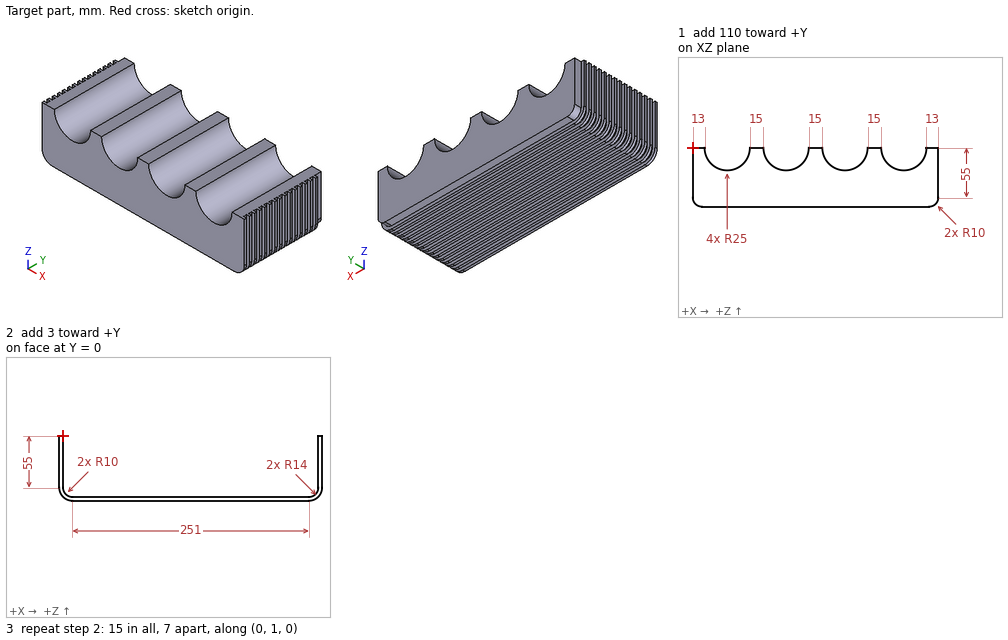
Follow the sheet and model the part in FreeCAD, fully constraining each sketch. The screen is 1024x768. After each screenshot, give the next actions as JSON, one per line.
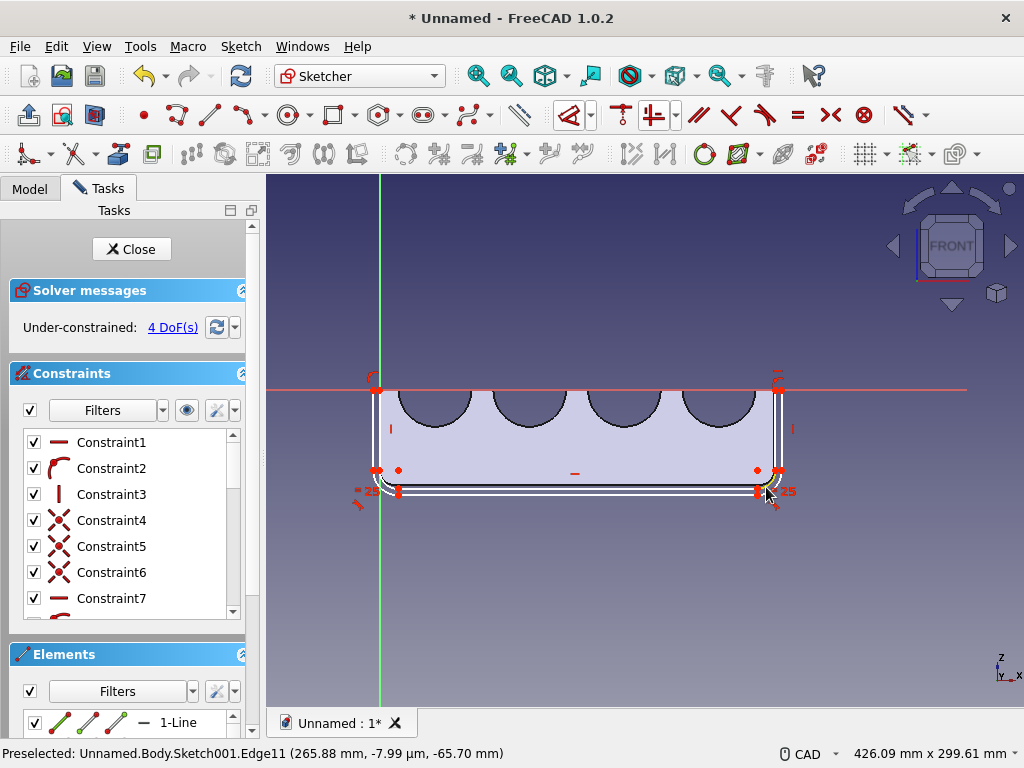
{"action": "scroll", "coordinate": [387, 493], "scroll_direction": "up", "scroll_amount": 4}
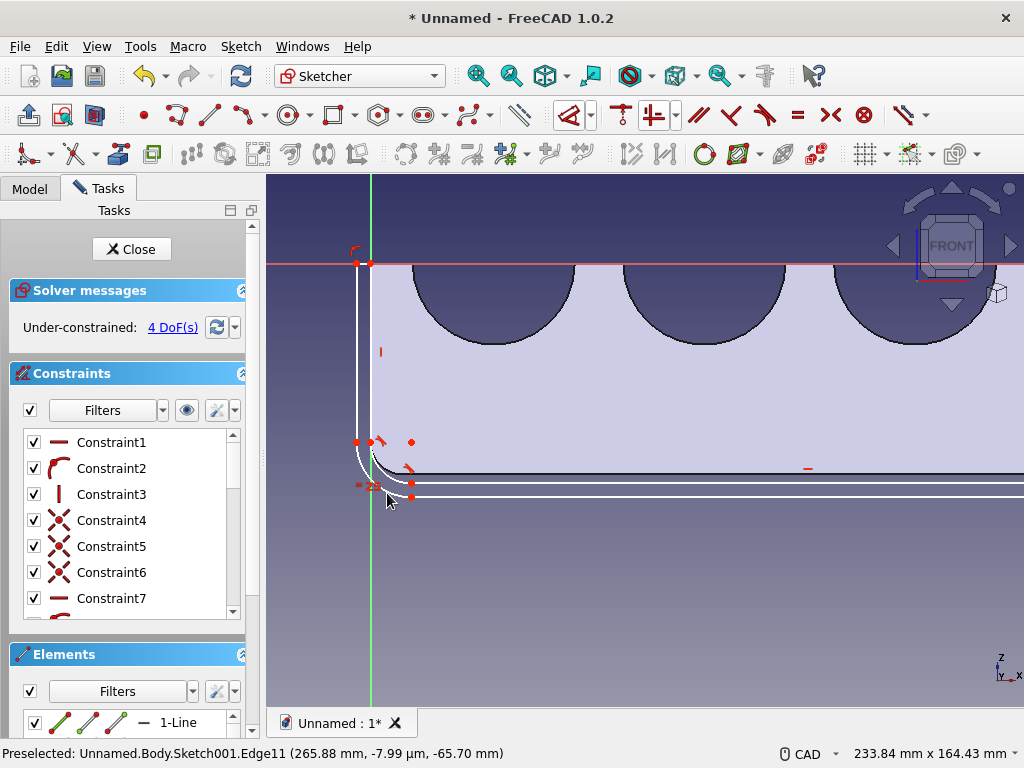
{"action": "left_click", "coordinate": [387, 491]}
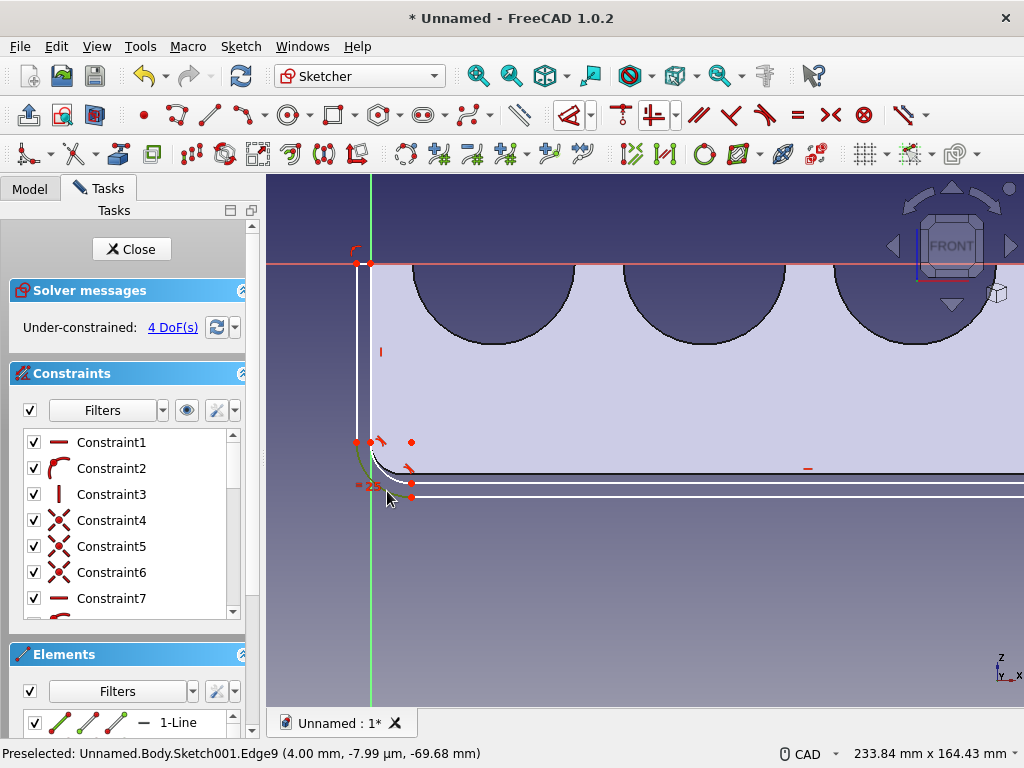
{"action": "key", "text": "k r"}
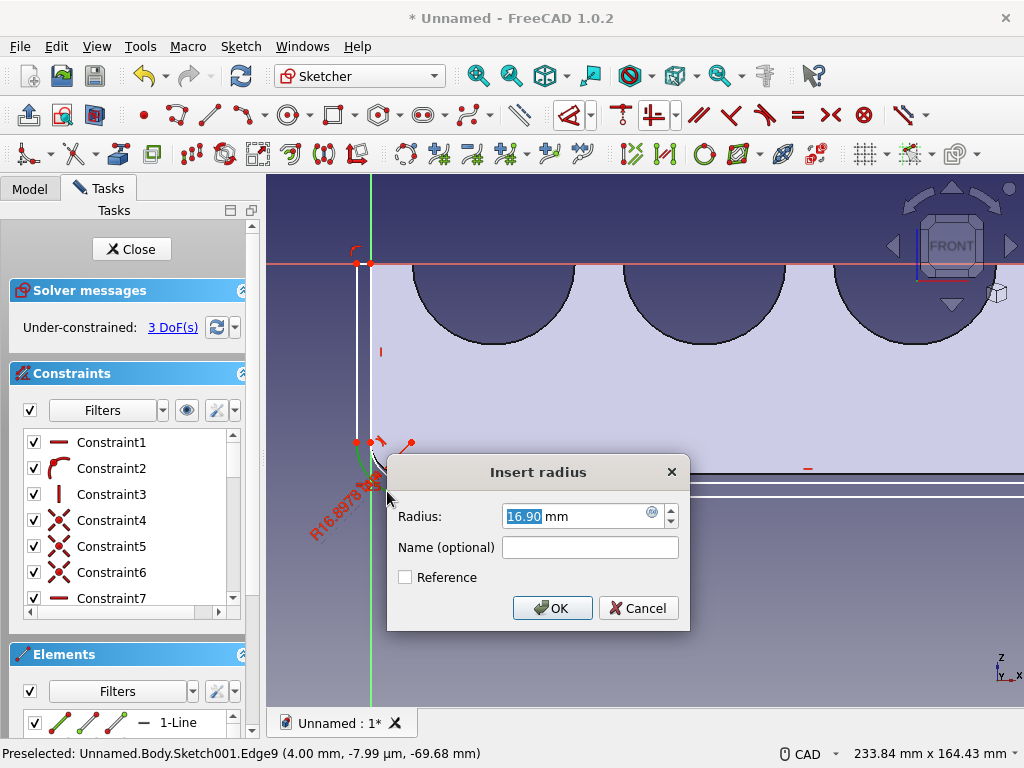
{"action": "type", "text": "14"}
{"action": "key", "text": "Return"}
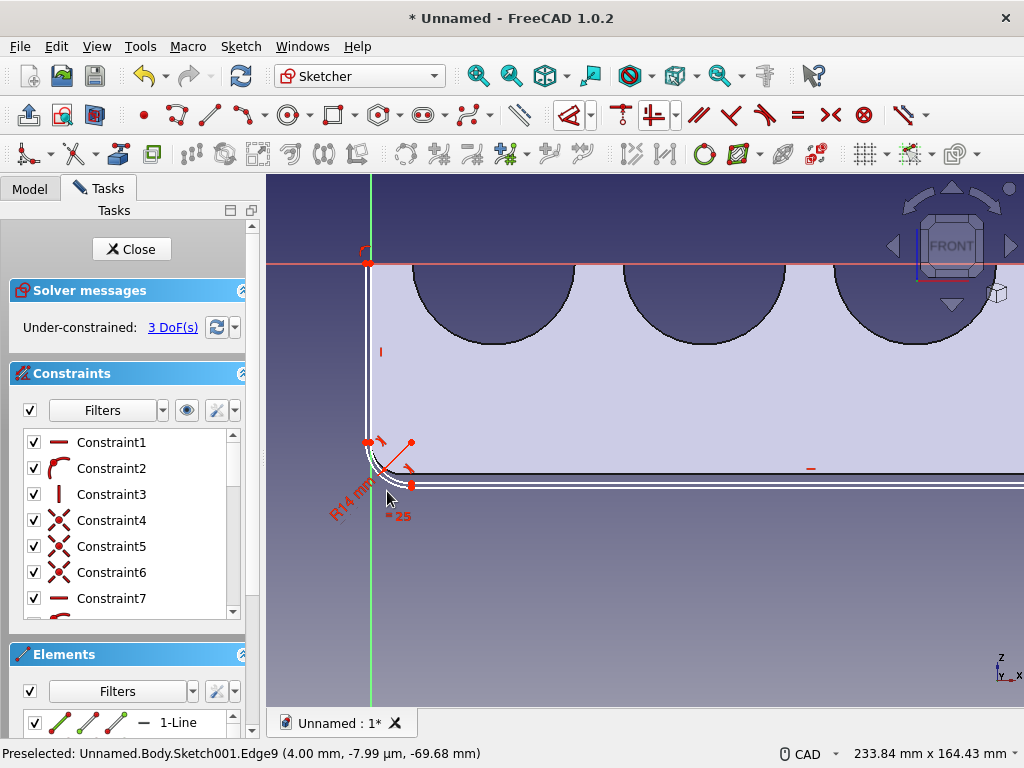
{"action": "scroll", "coordinate": [373, 455], "scroll_direction": "up", "scroll_amount": 6}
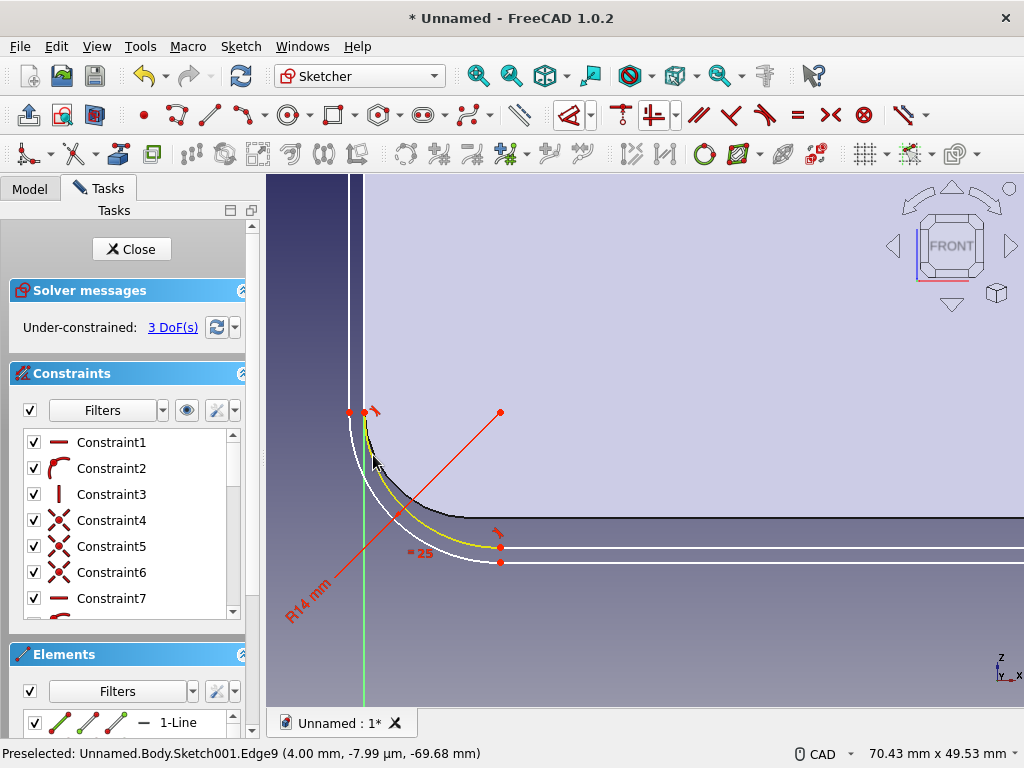
{"action": "left_click", "coordinate": [371, 454]}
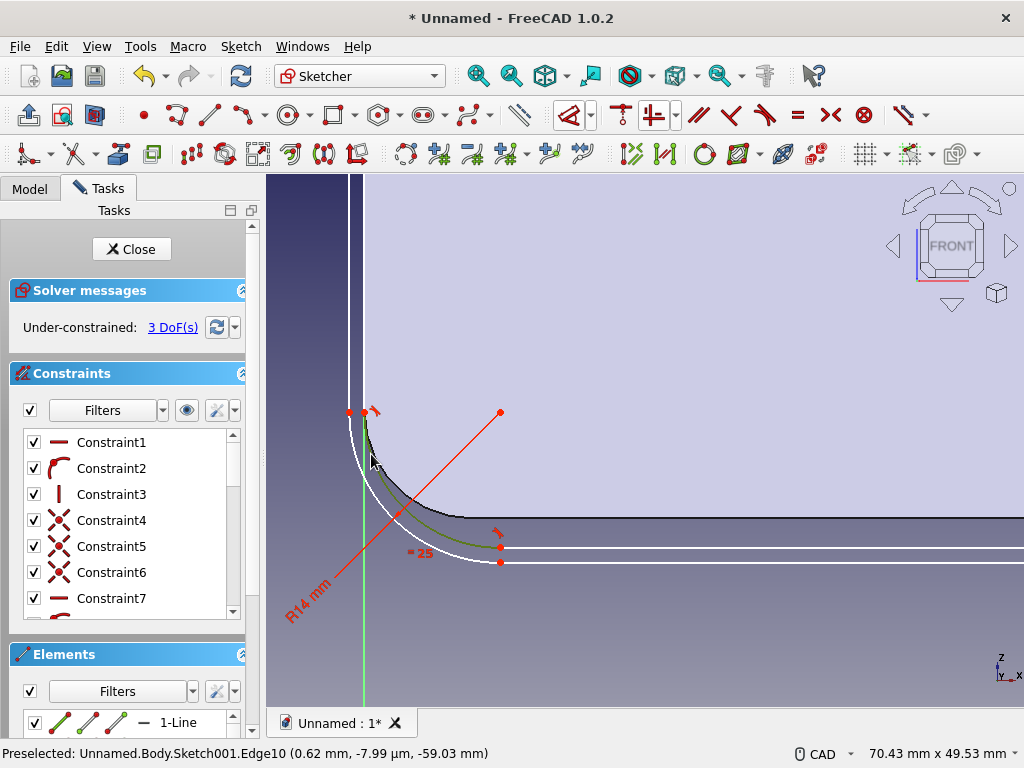
{"action": "key", "text": "k r"}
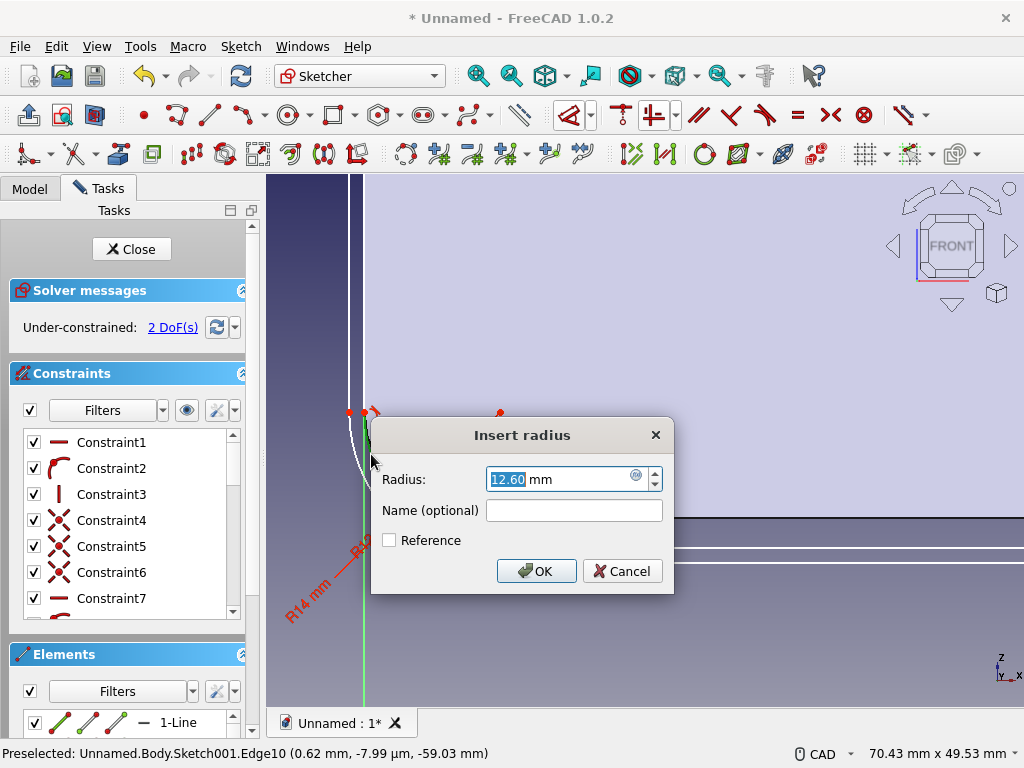
{"action": "type", "text": "10"}
{"action": "key", "text": "Return"}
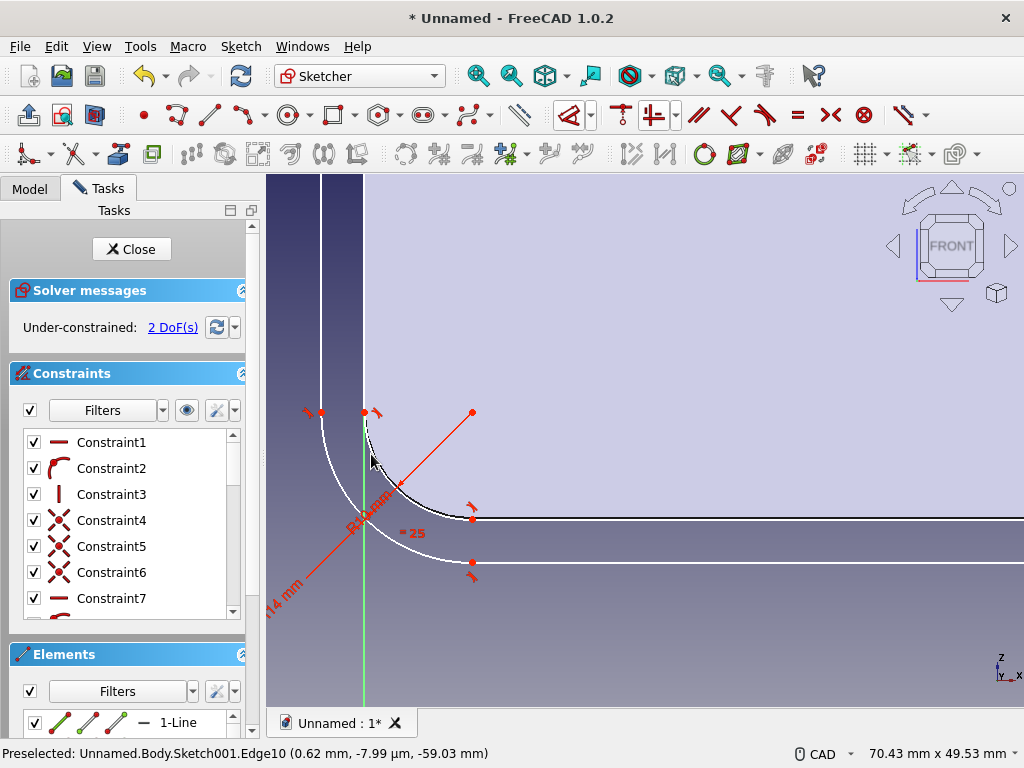
{"action": "scroll", "coordinate": [381, 480], "scroll_direction": "down", "scroll_amount": 10}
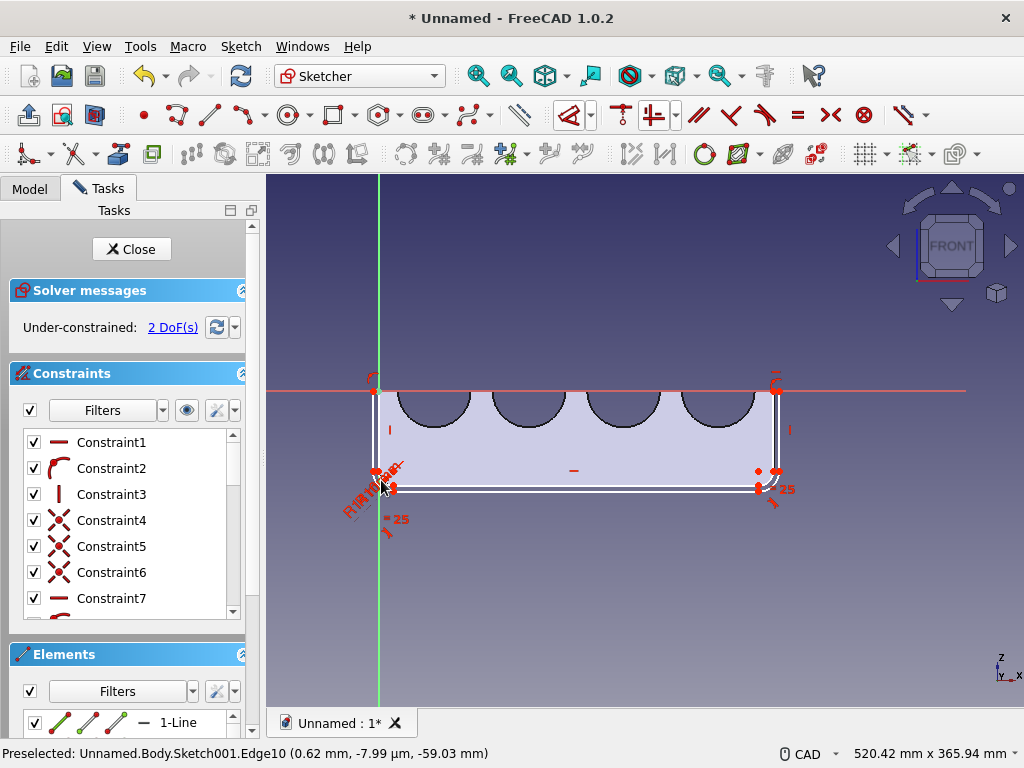
{"action": "scroll", "coordinate": [373, 447], "scroll_direction": "up", "scroll_amount": 5}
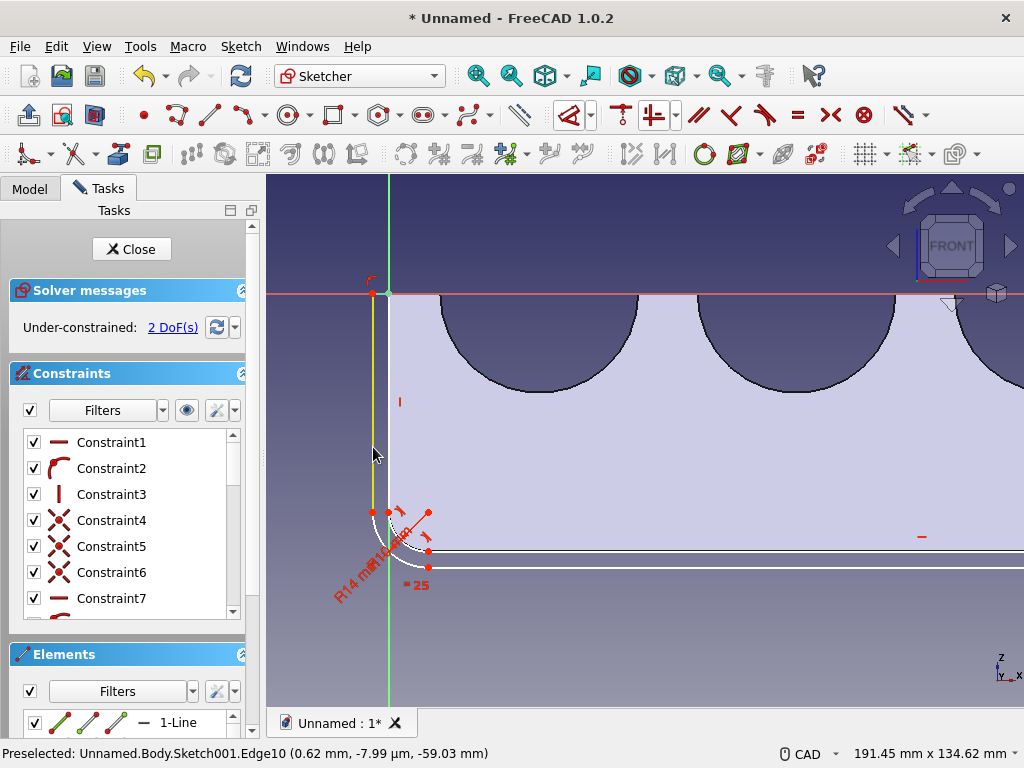
{"action": "left_click", "coordinate": [373, 447]}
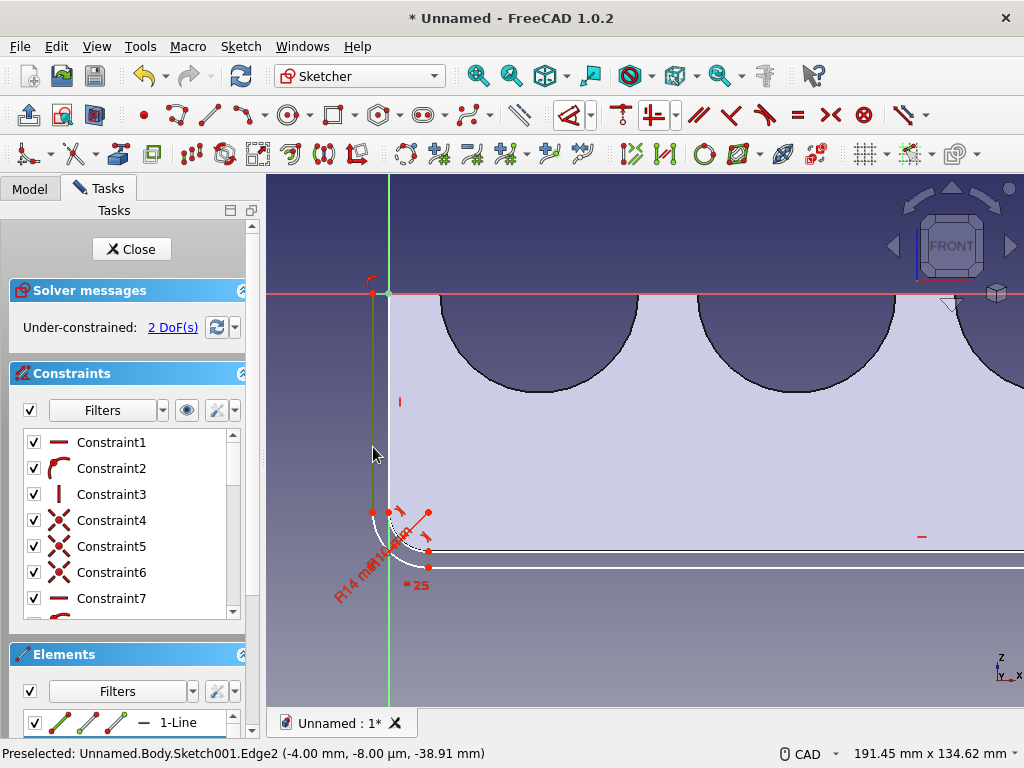
{"action": "key", "text": "i"}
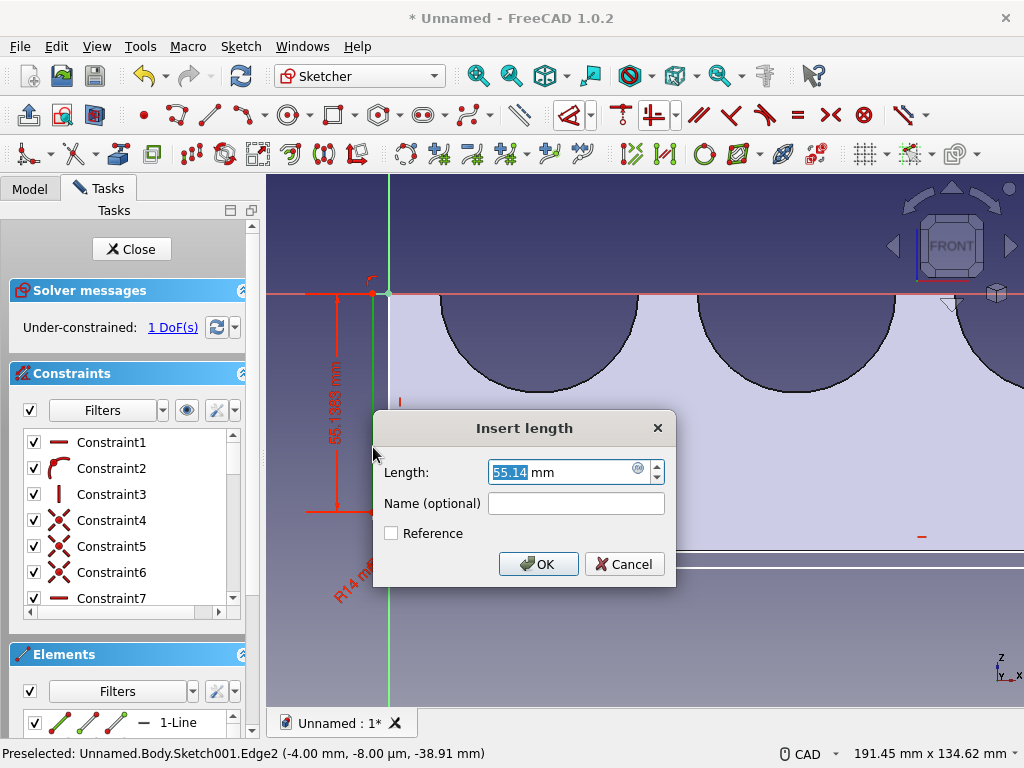
{"action": "type", "text": "55"}
{"action": "key", "text": "Return"}